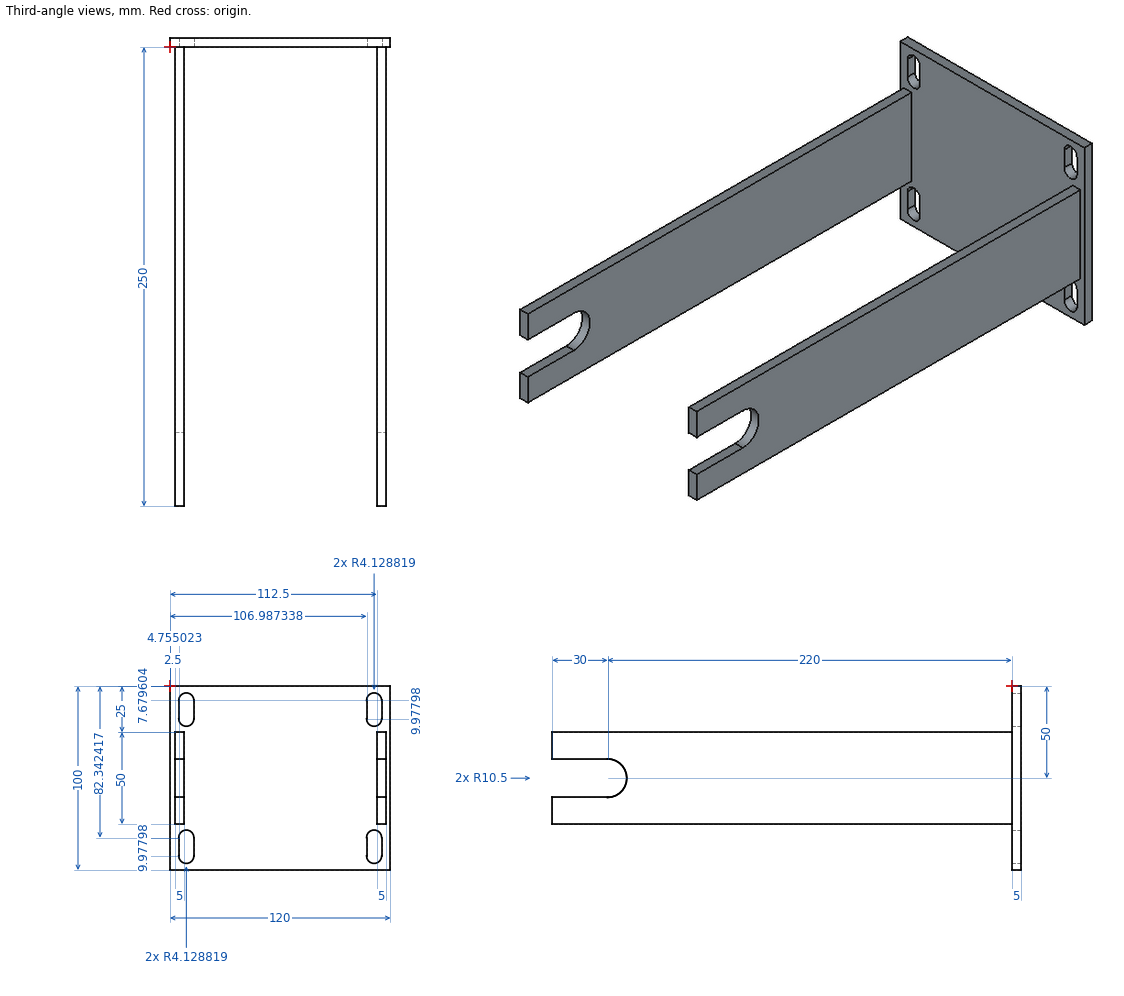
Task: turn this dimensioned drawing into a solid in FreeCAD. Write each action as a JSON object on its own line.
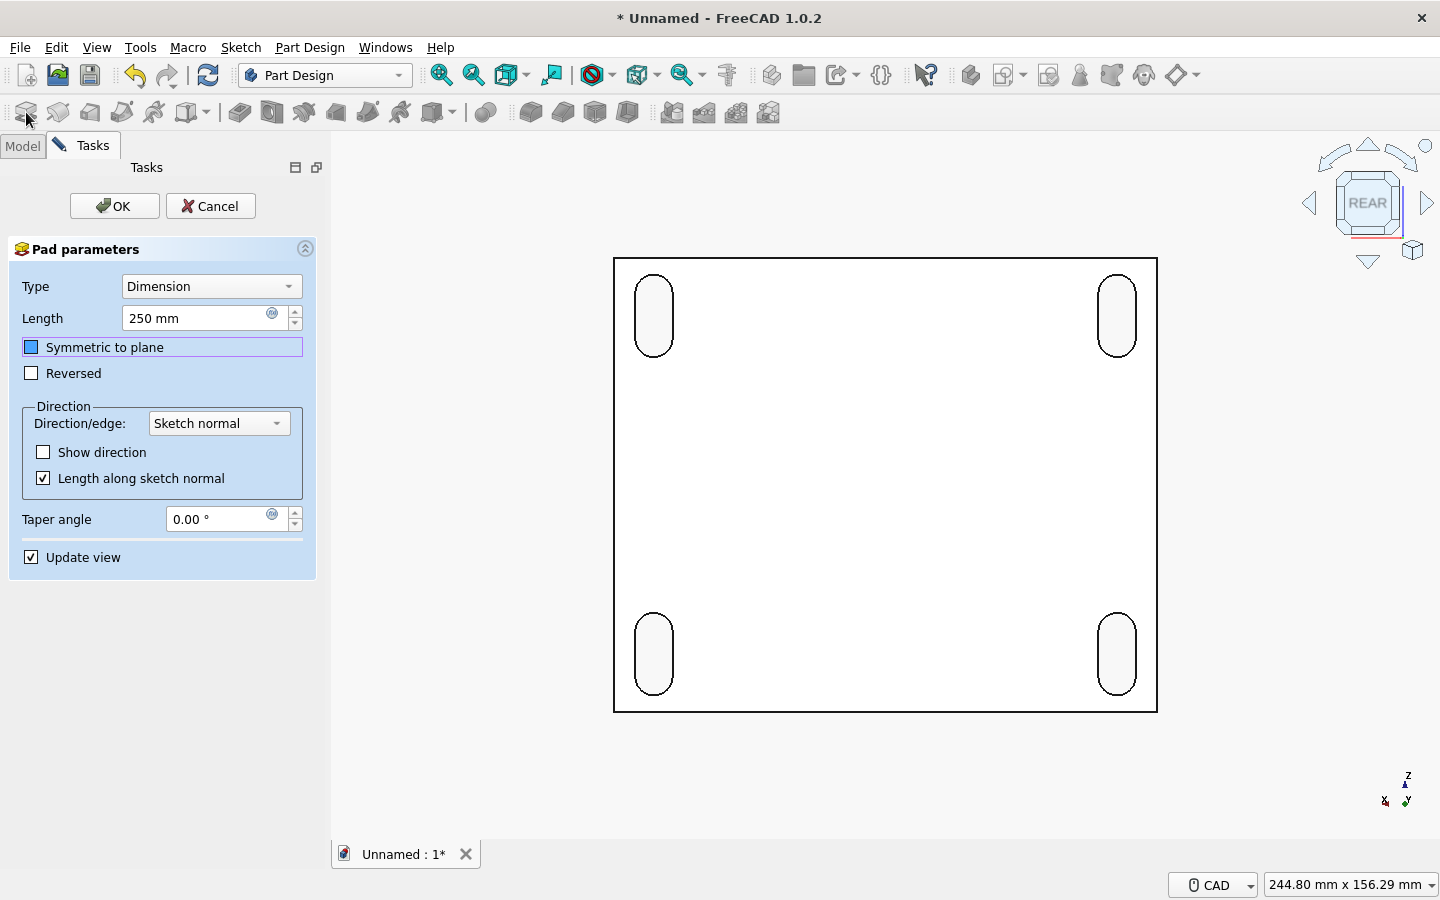
{"action": "left_click", "coordinate": [115, 206]}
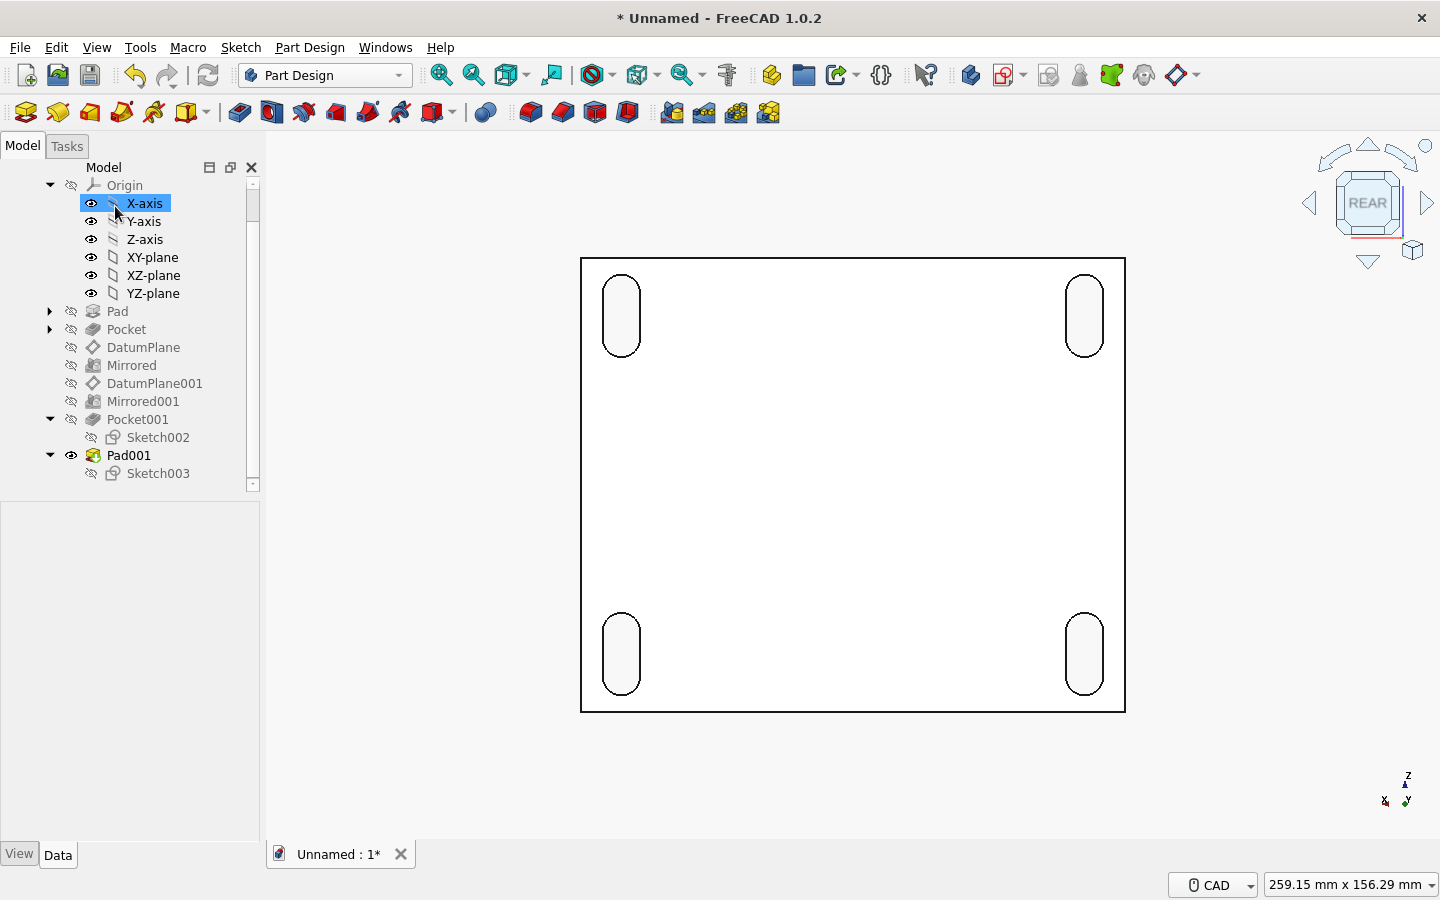
{"action": "key", "text": "6"}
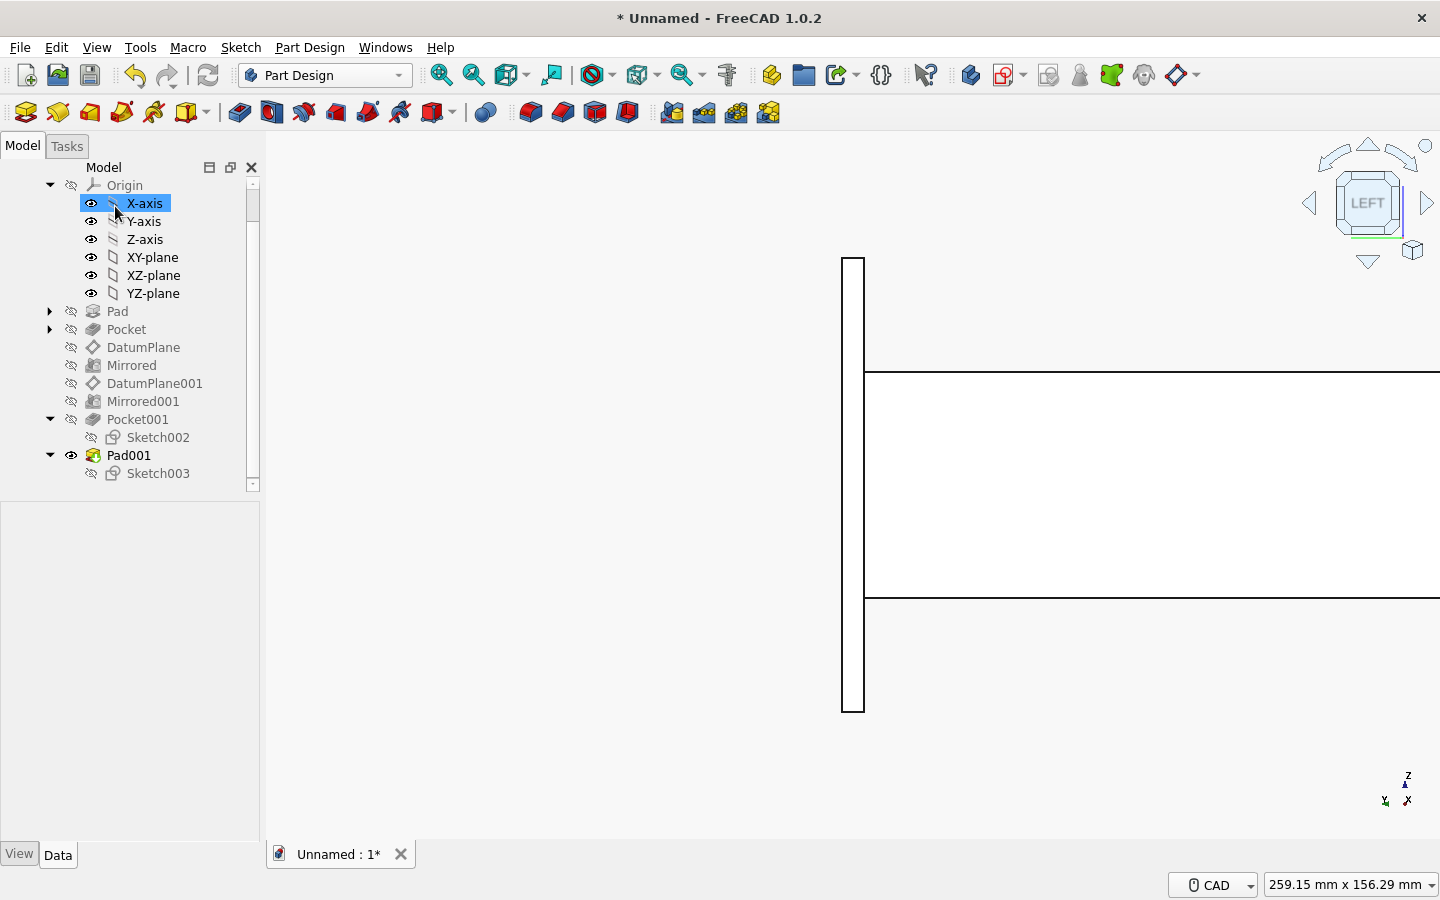
{"action": "left_click", "coordinate": [442, 76]}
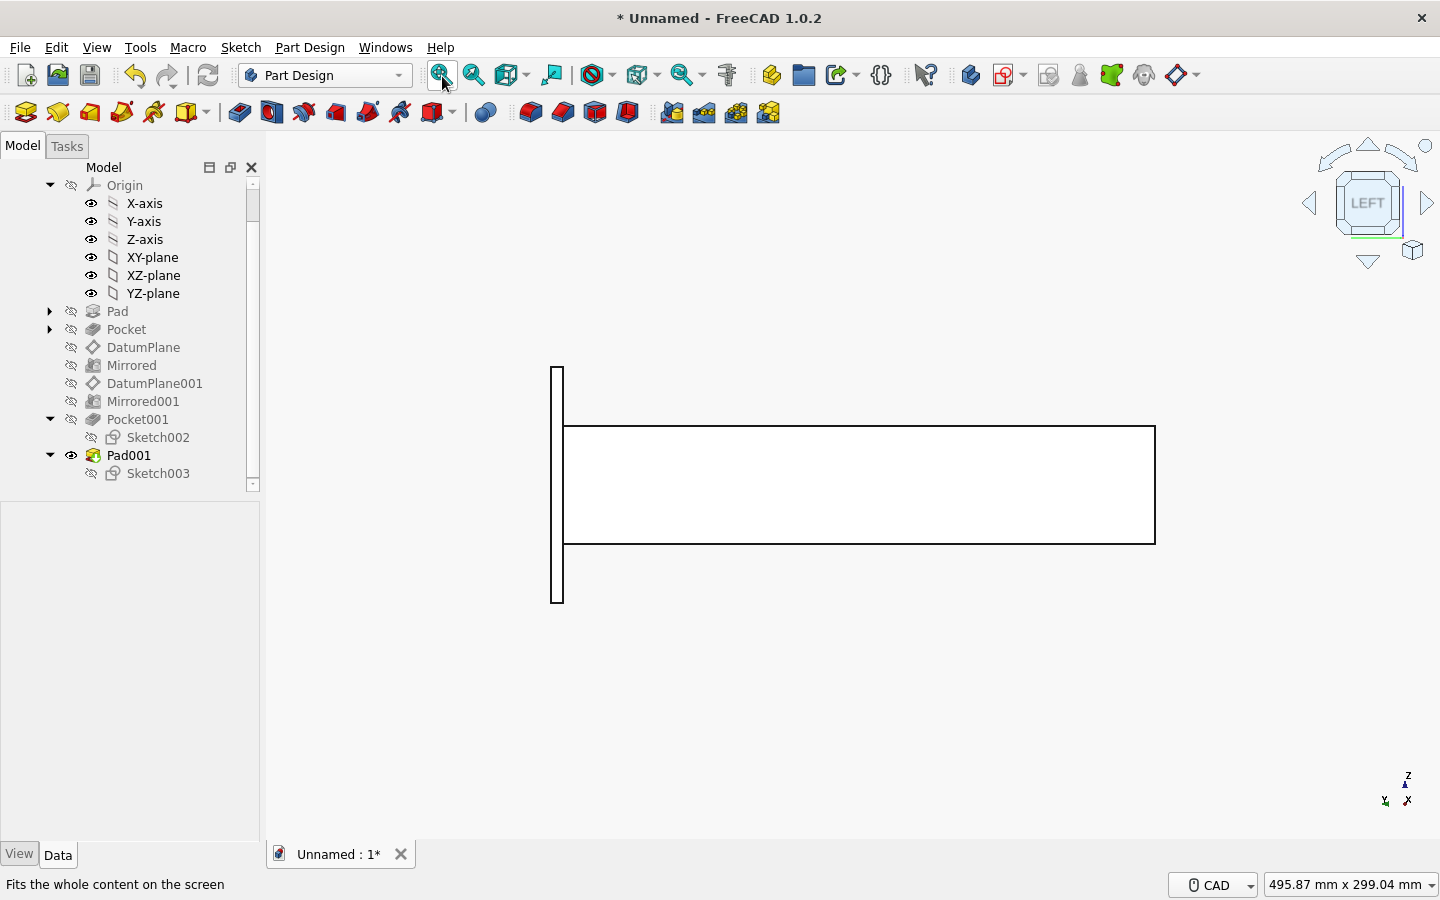
{"action": "left_click", "coordinate": [774, 484]}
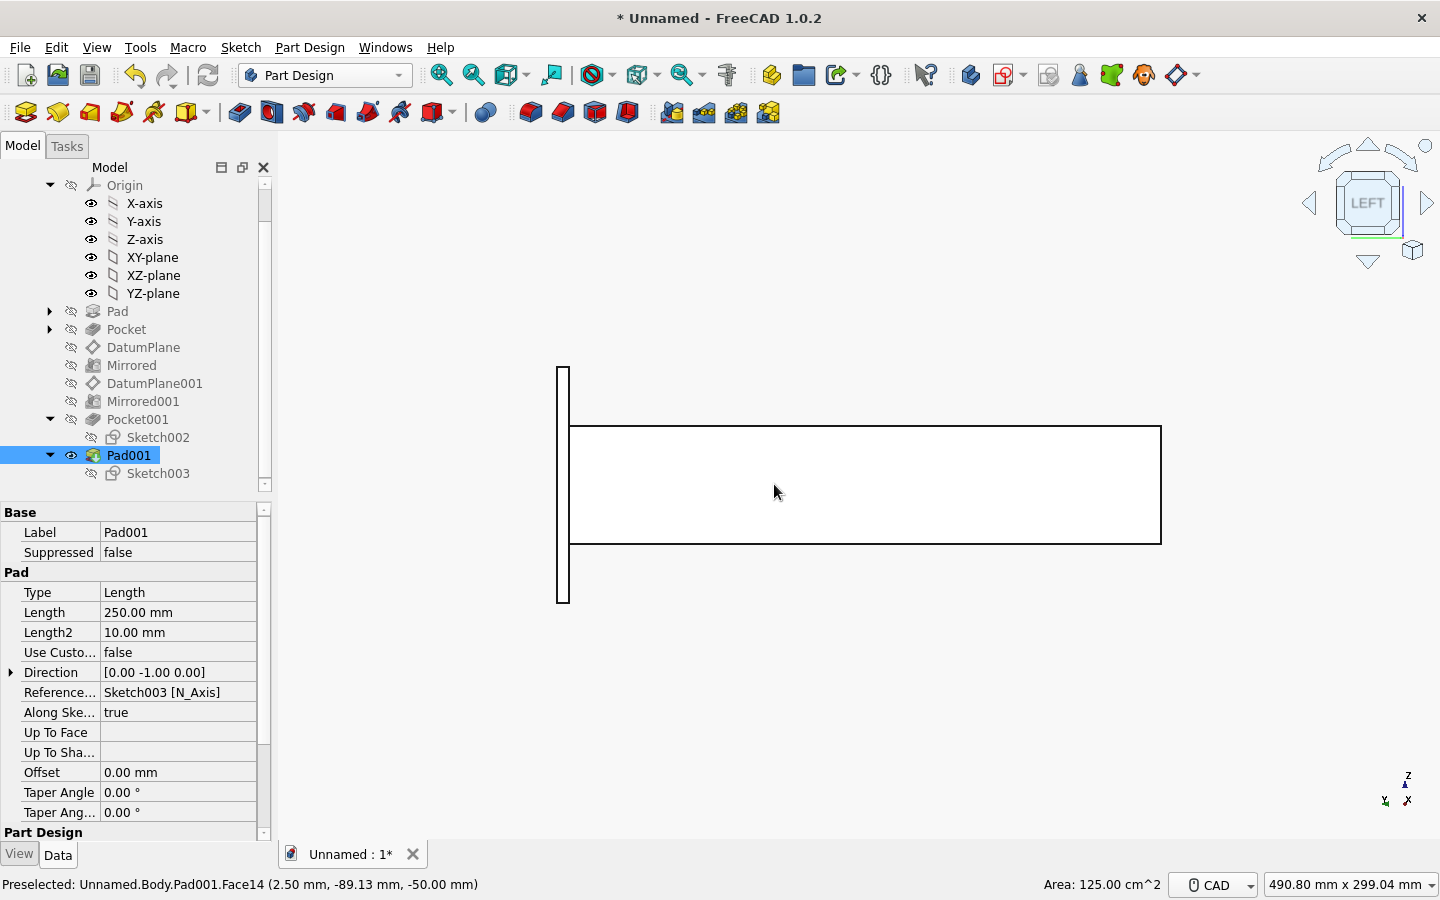
{"action": "left_click", "coordinate": [1004, 76]}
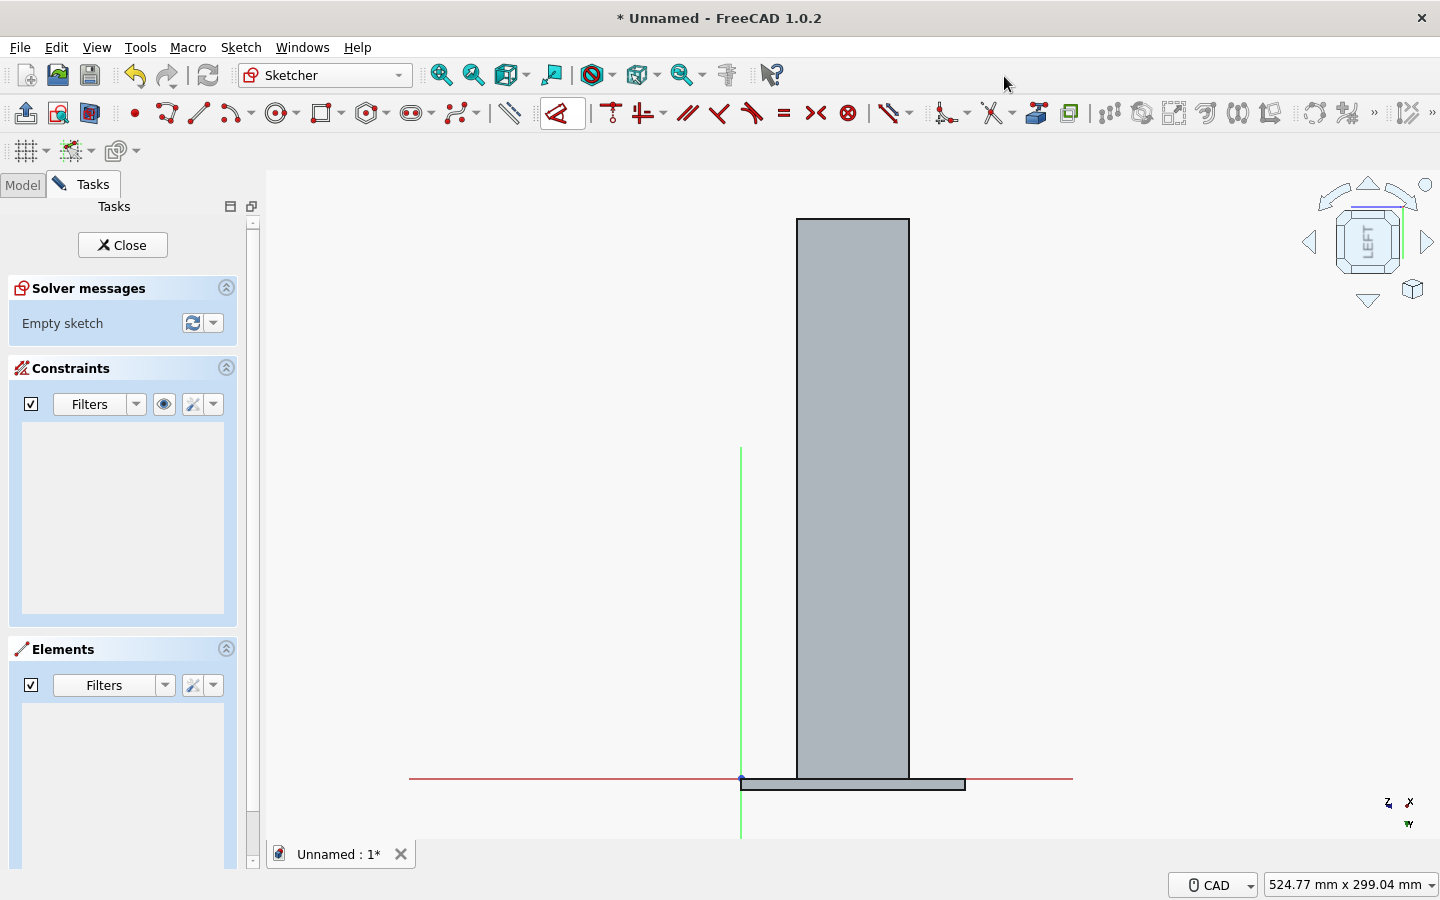
{"action": "key", "text": "q s"}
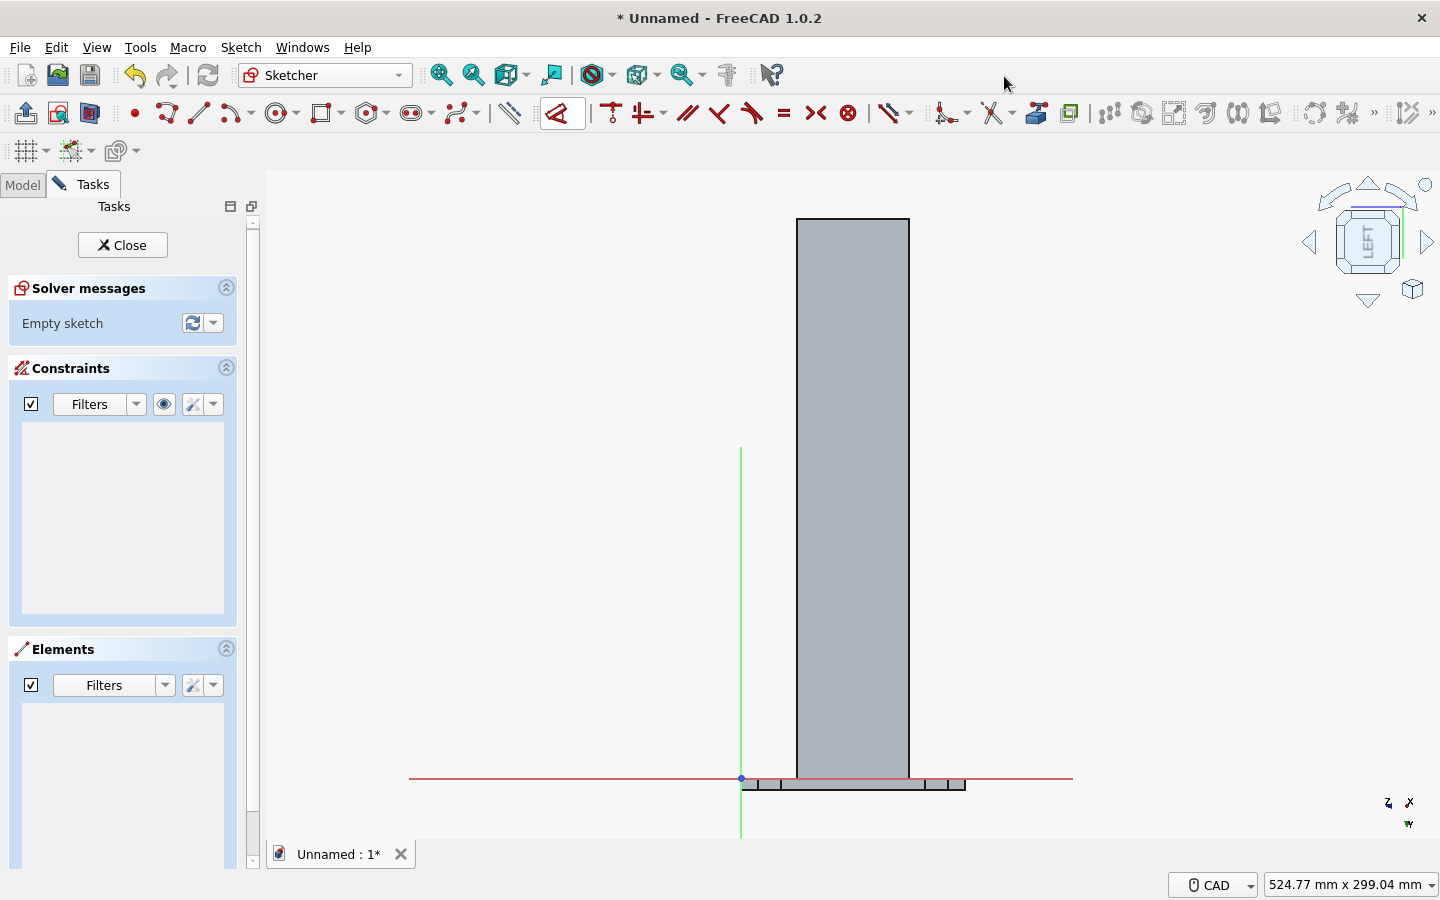
{"action": "scroll", "coordinate": [784, 504], "scroll_direction": "down", "scroll_amount": 5}